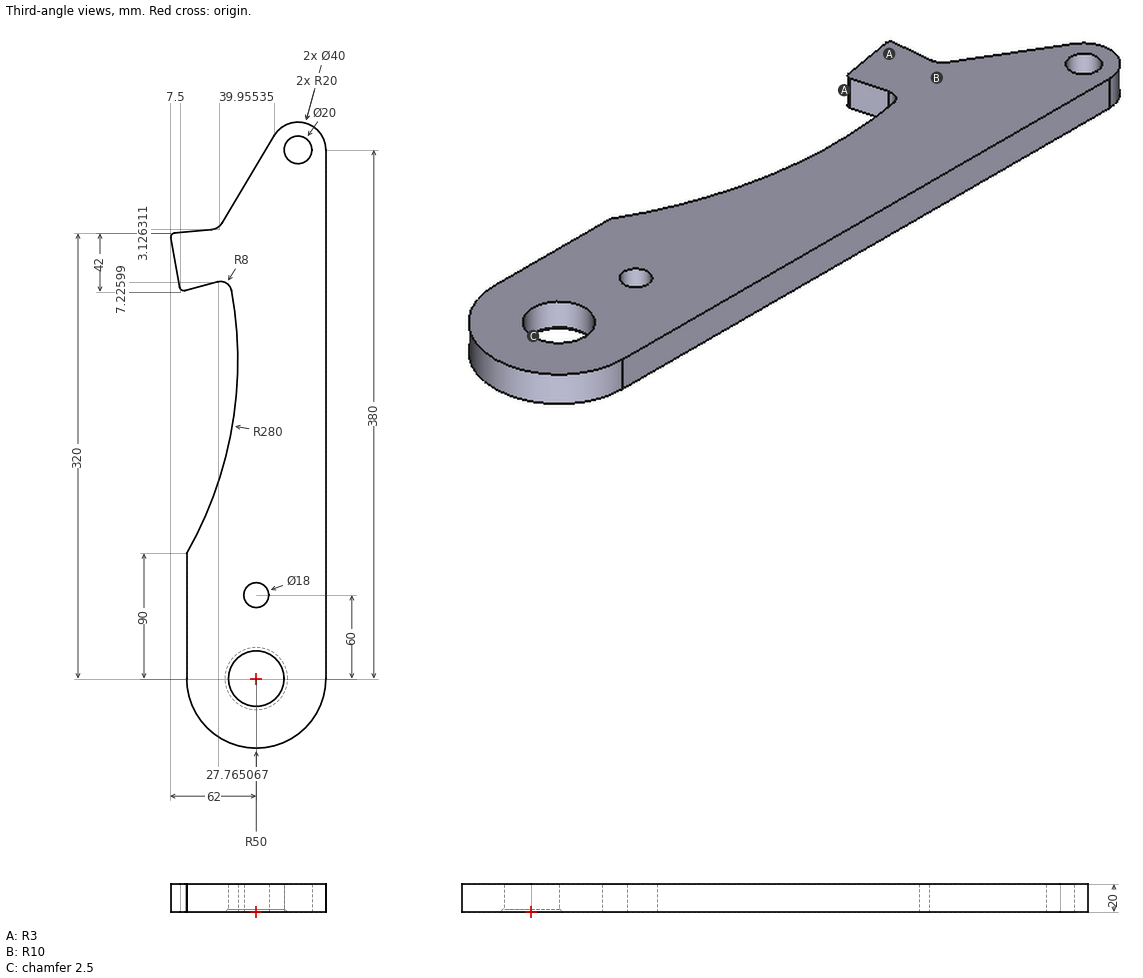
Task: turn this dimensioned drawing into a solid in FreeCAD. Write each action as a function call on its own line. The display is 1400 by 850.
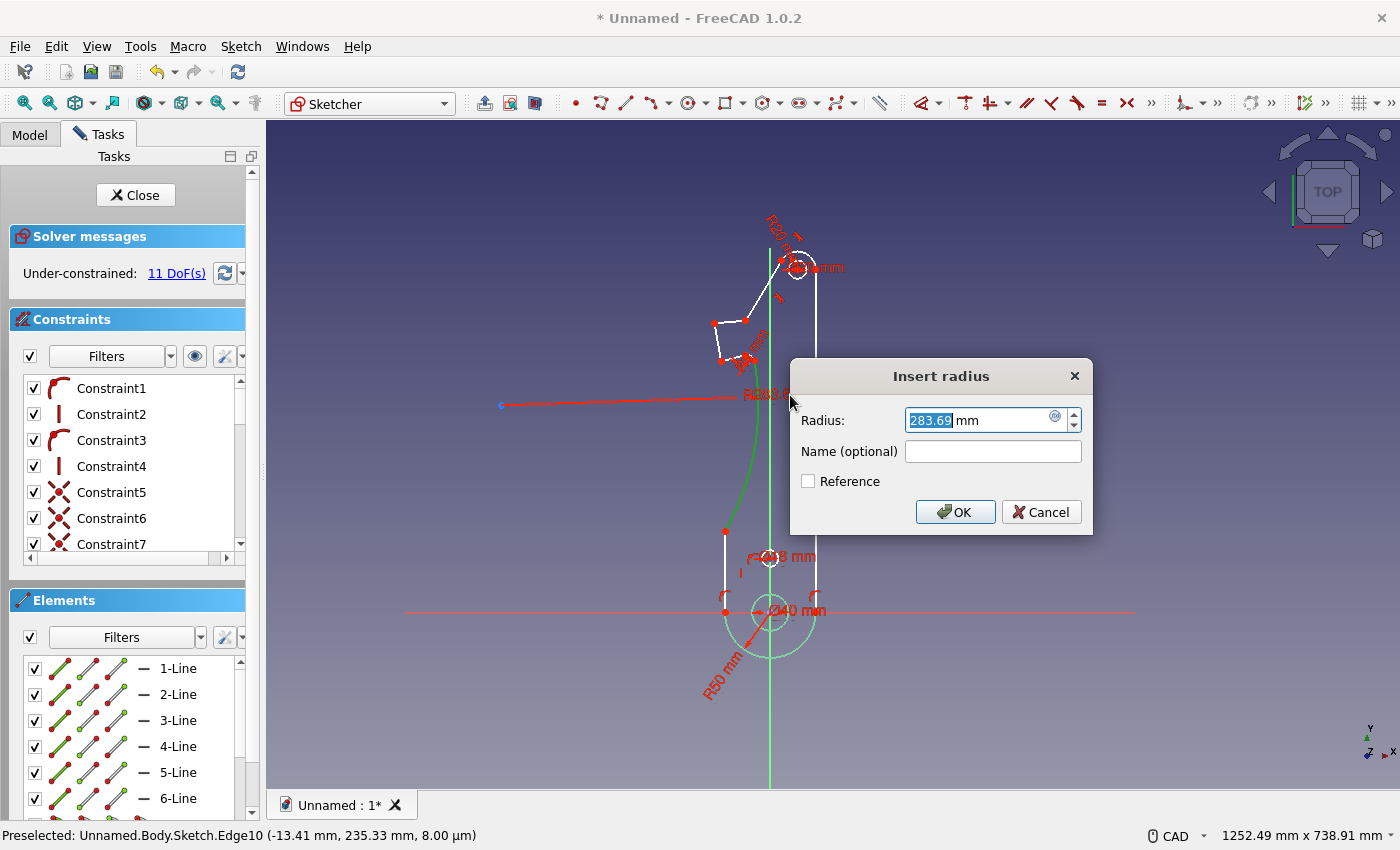
text(280)
key(Return)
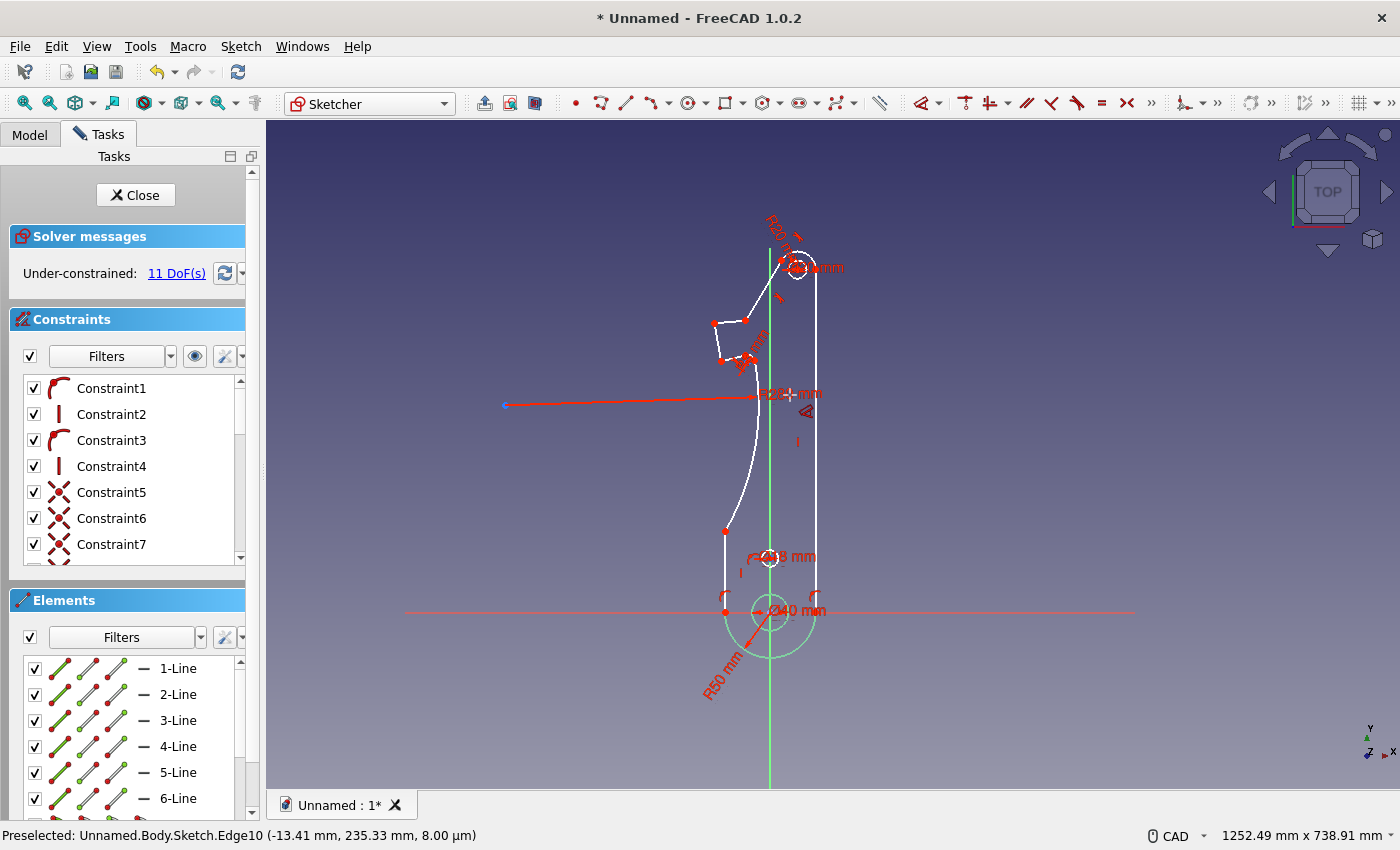
click(725, 556)
click(691, 572)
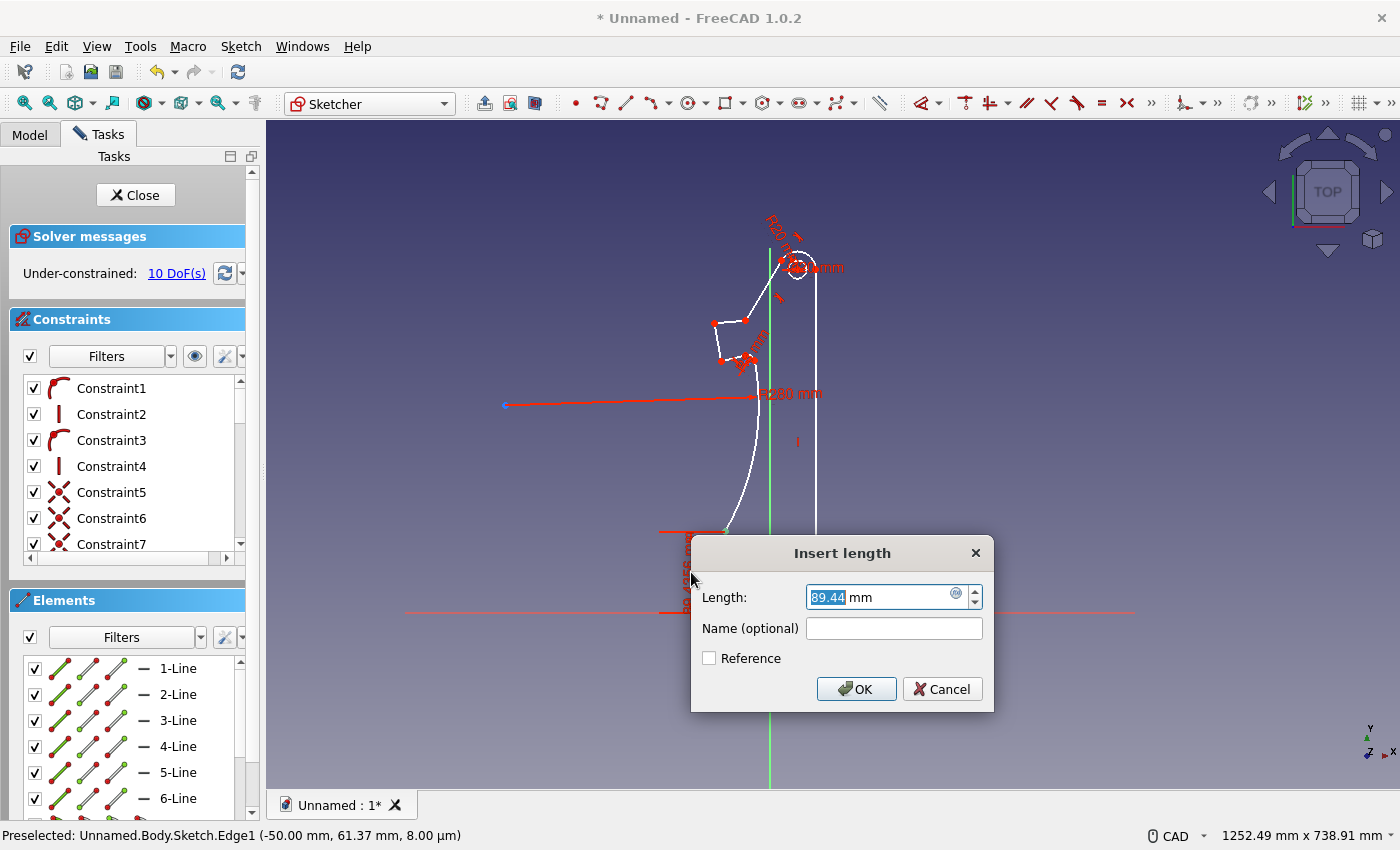
text(90)
key(Return)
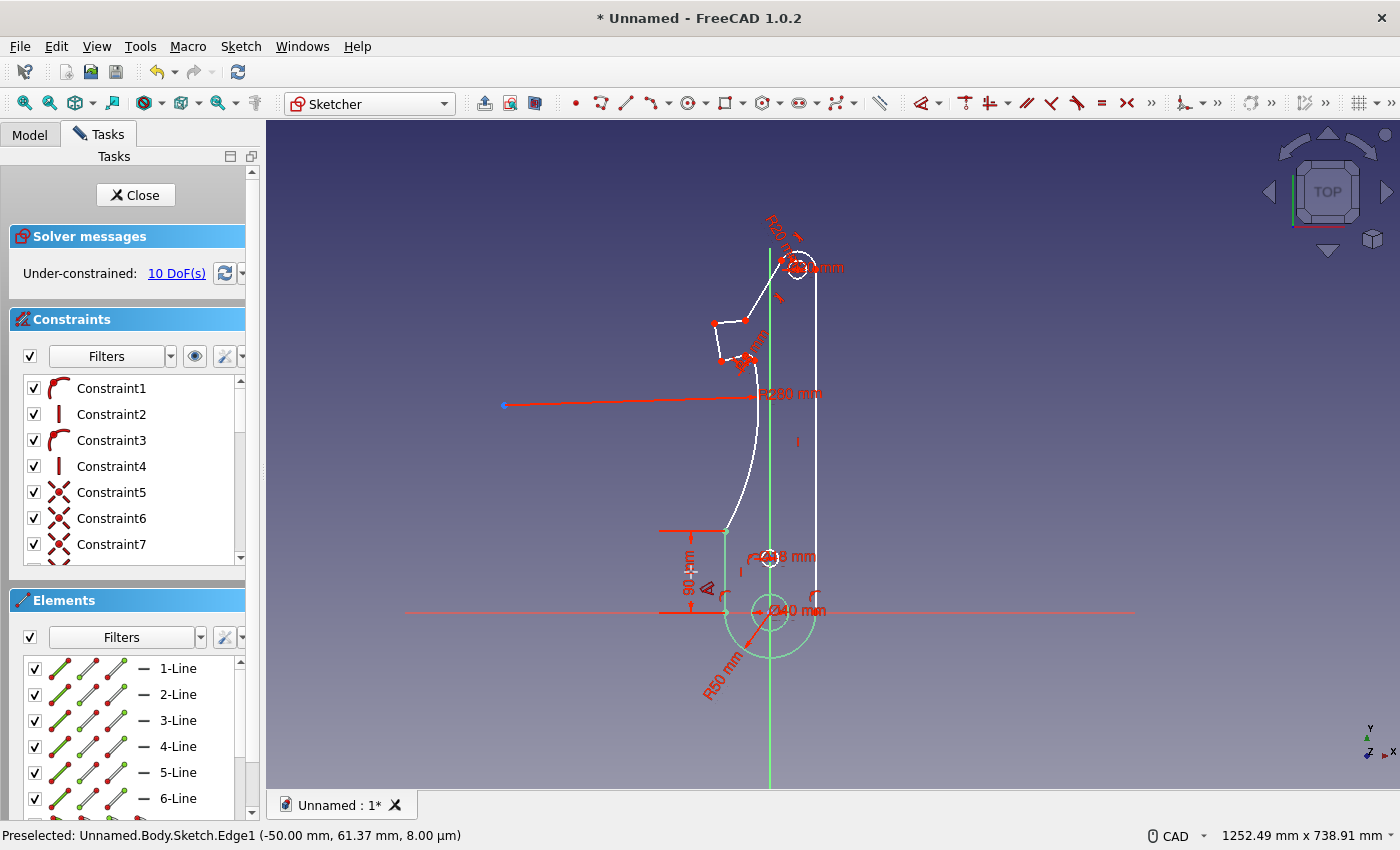
click(770, 559)
click(852, 586)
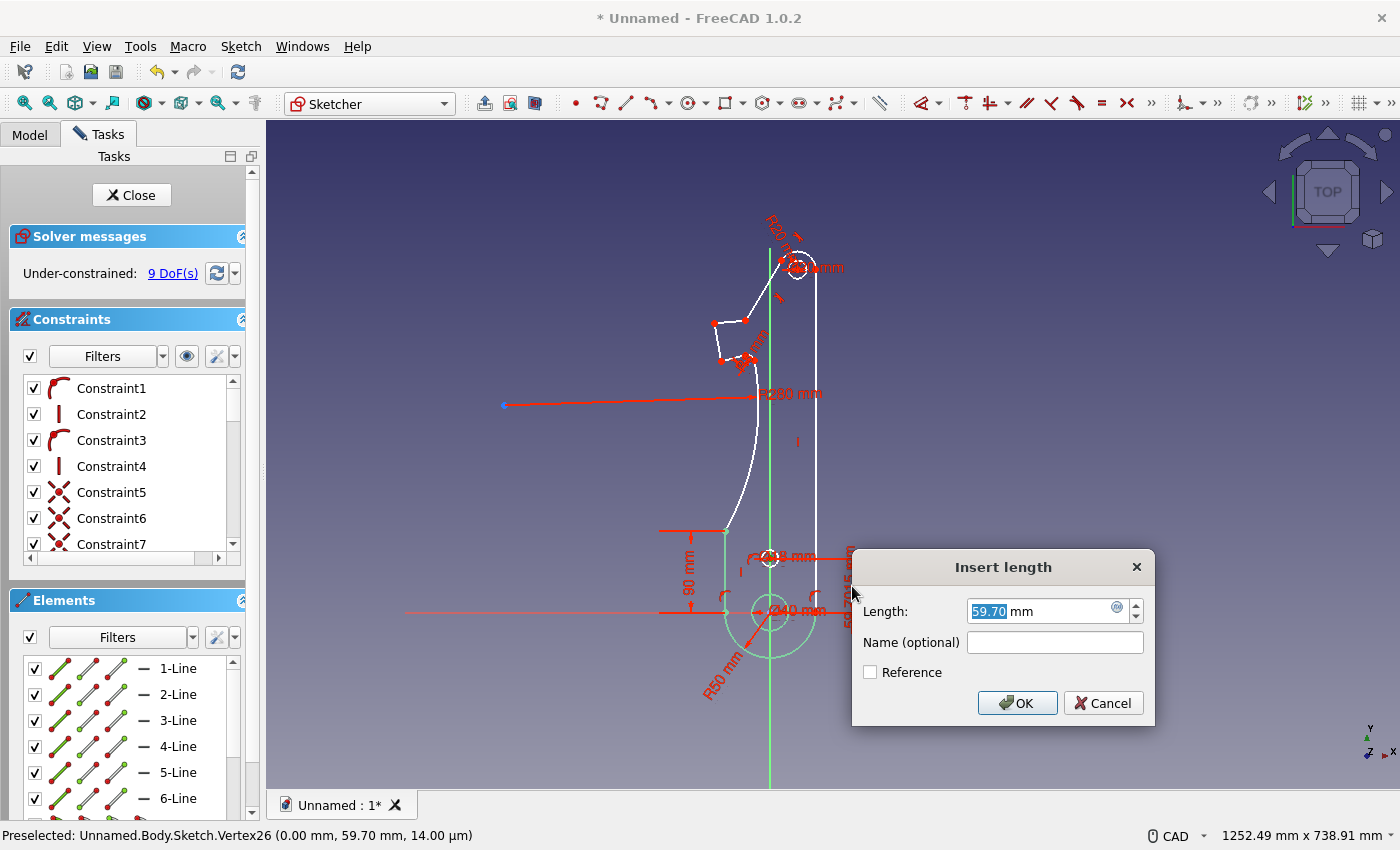
text(60)
key(Return)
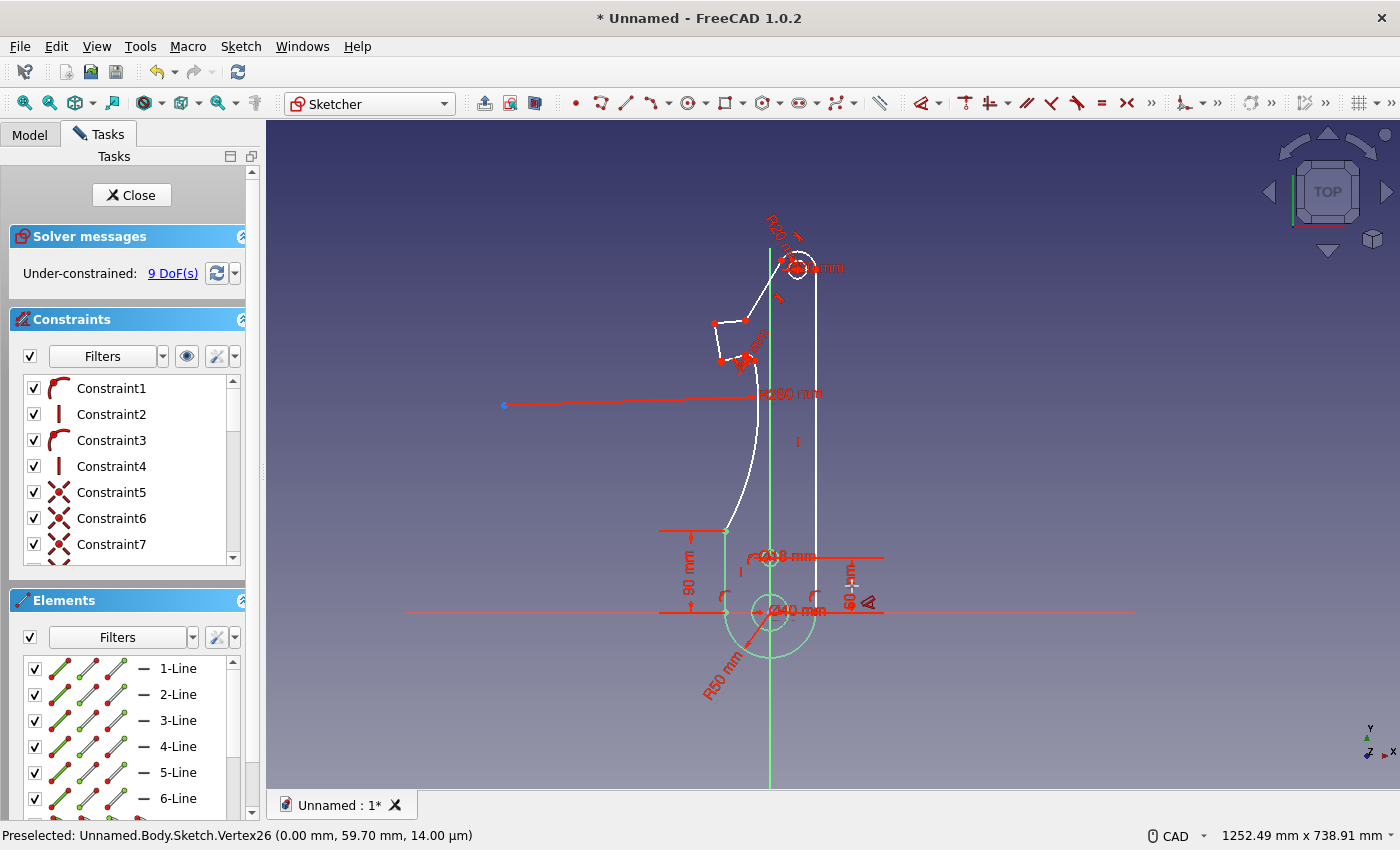
click(816, 510)
click(850, 441)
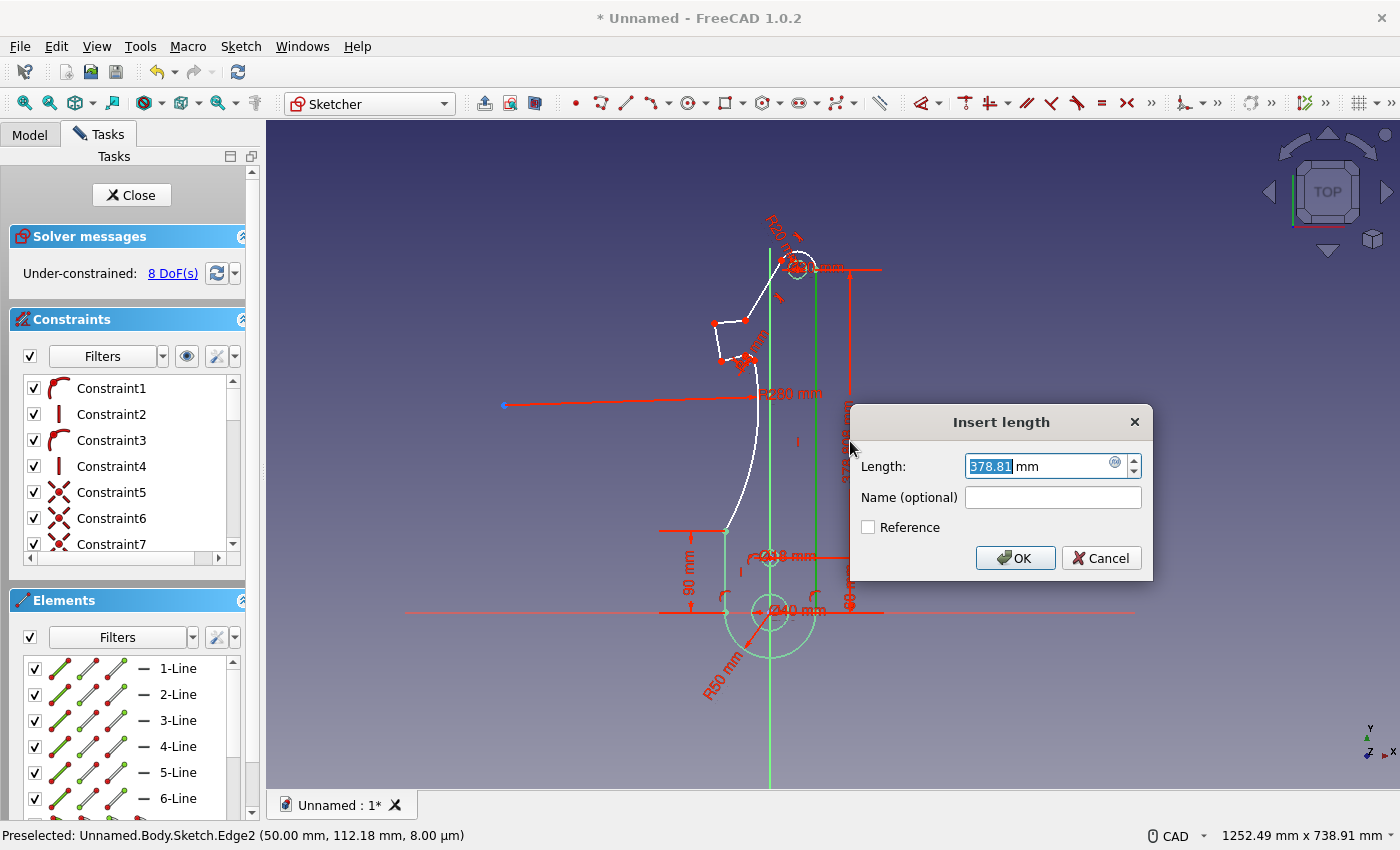
text(380)
key(Return)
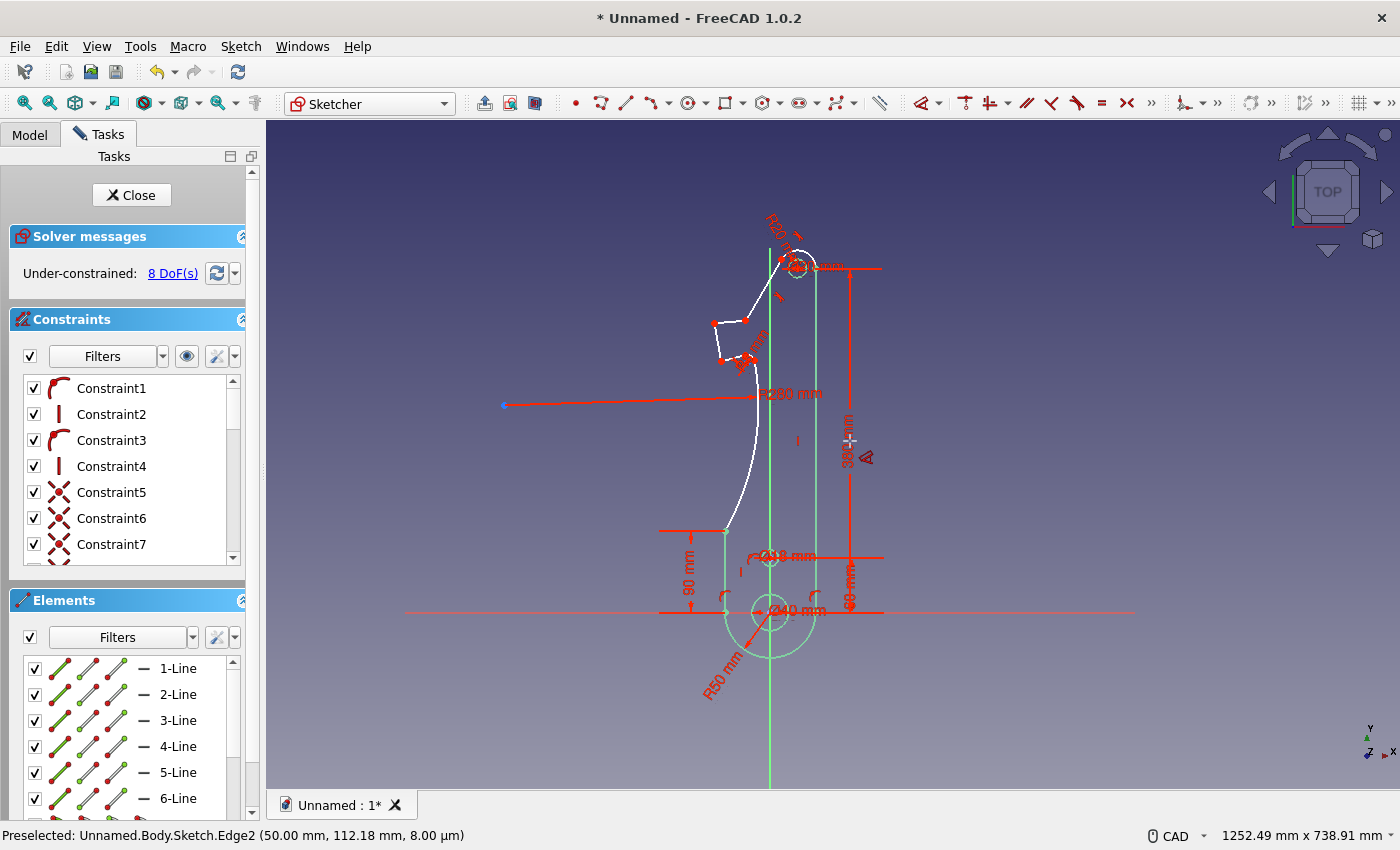
click(714, 323)
click(723, 647)